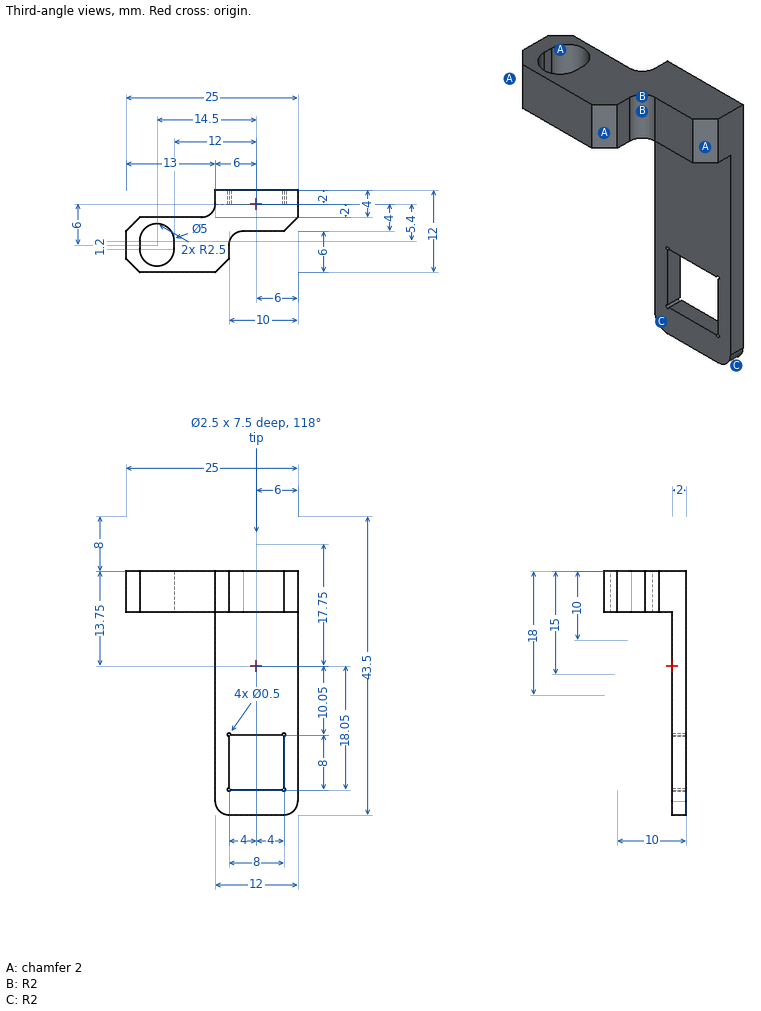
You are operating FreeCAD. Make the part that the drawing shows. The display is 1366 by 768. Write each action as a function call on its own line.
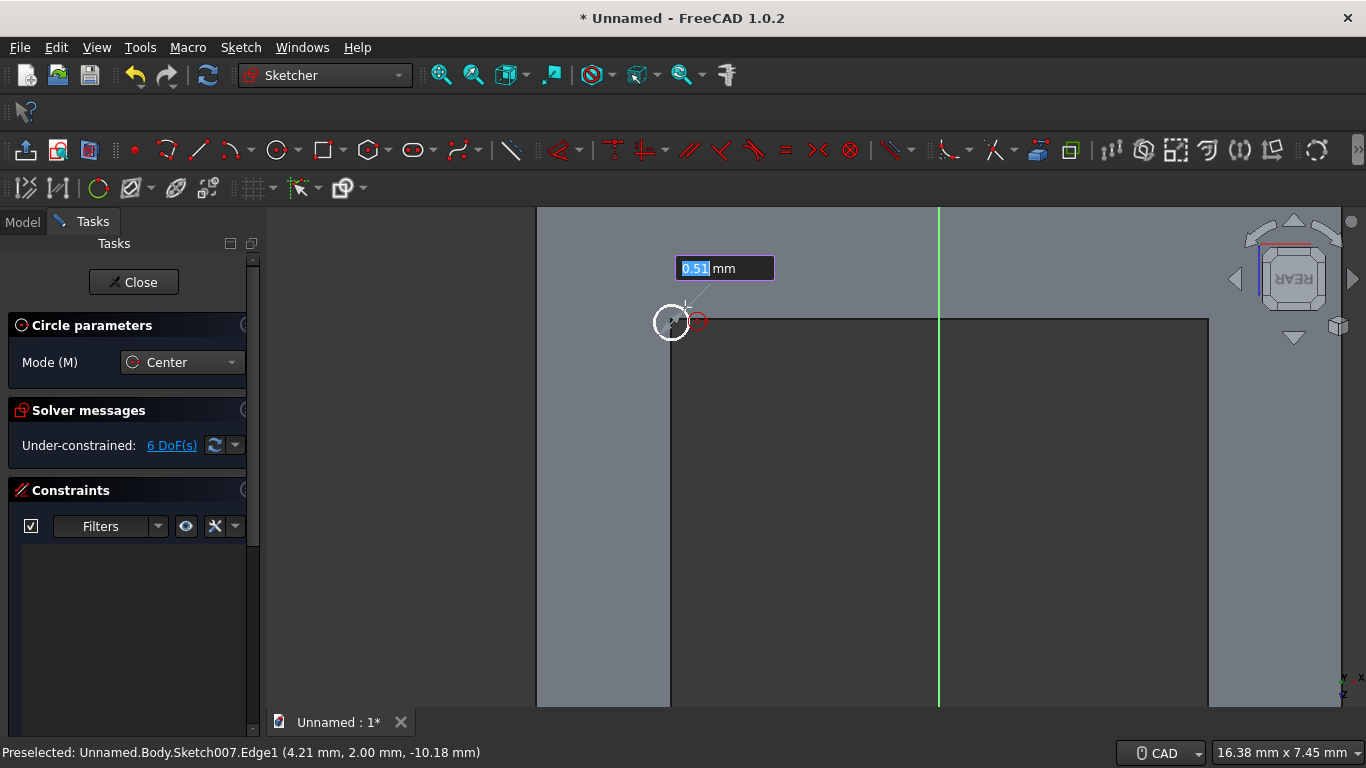
click(683, 307)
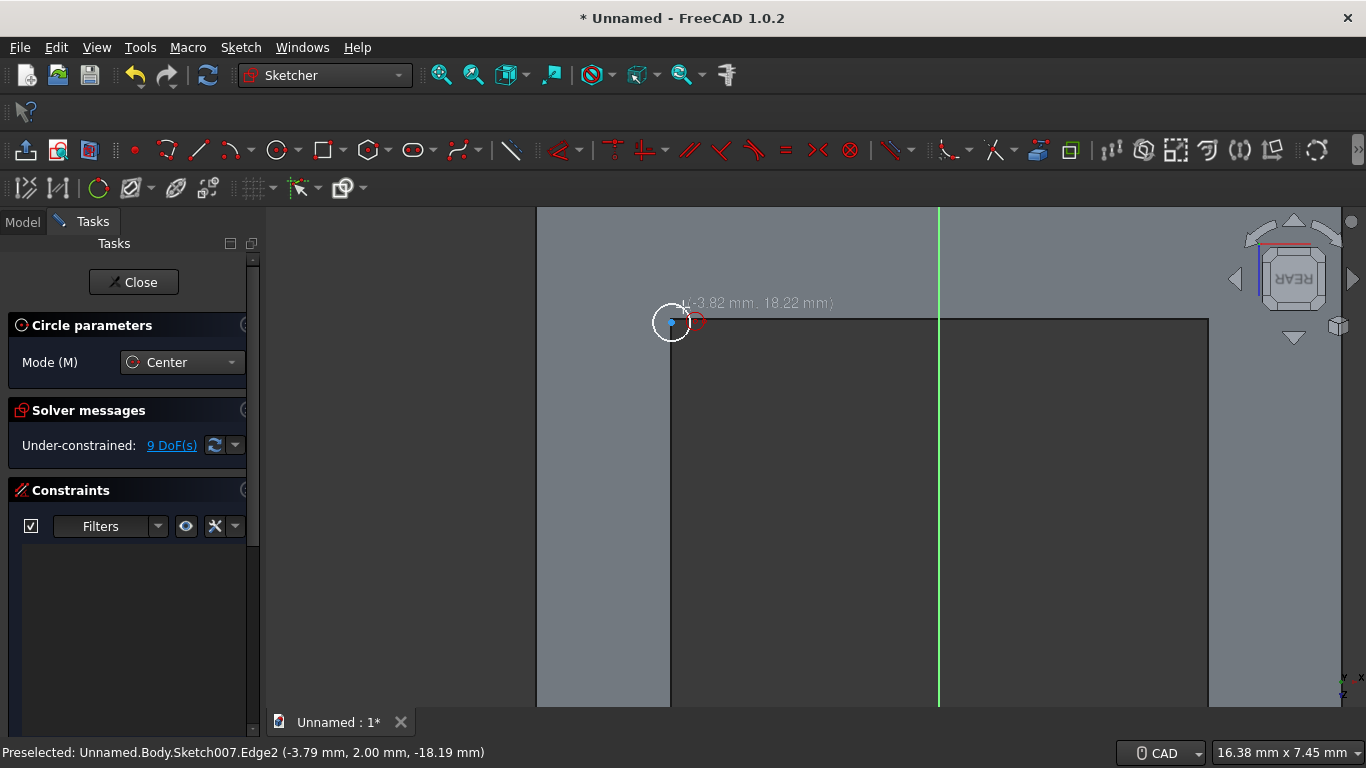
scroll(685, 306, down, 7)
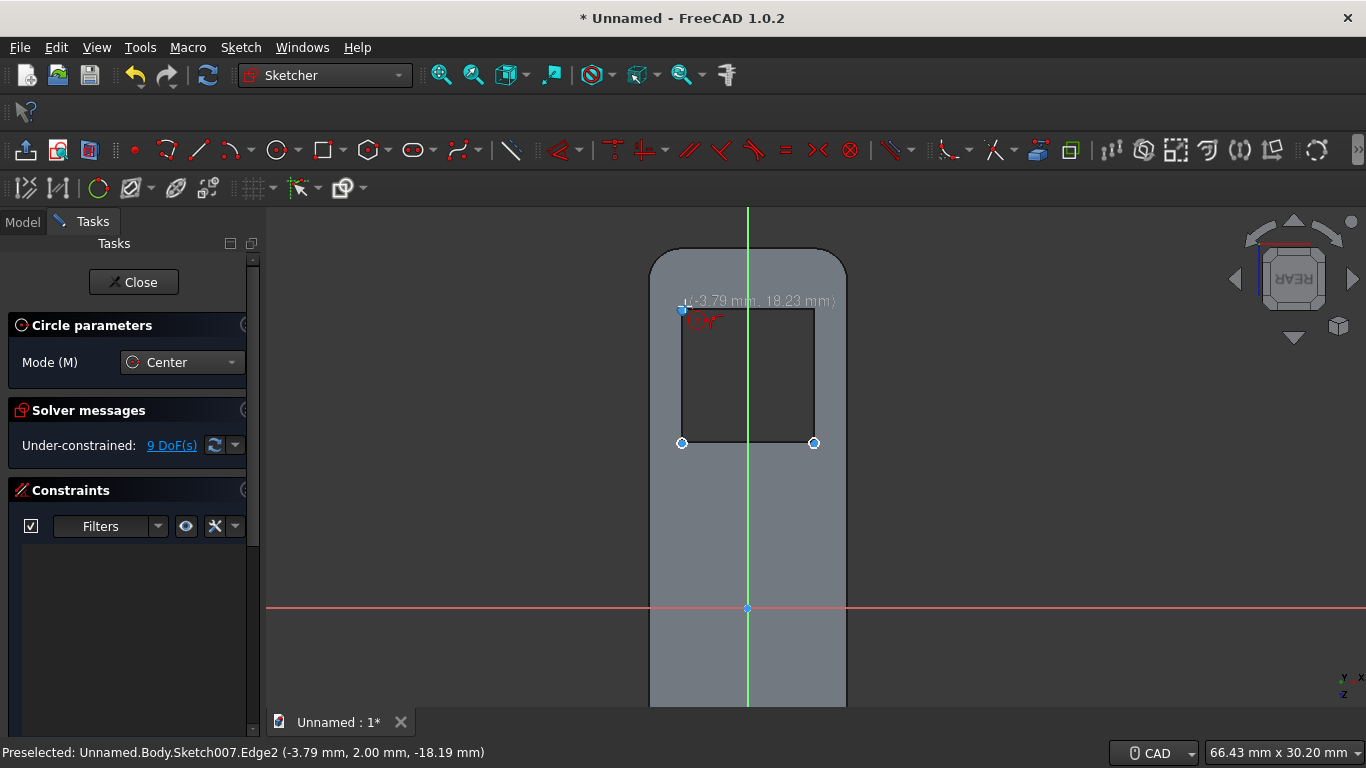
scroll(814, 309, up, 9)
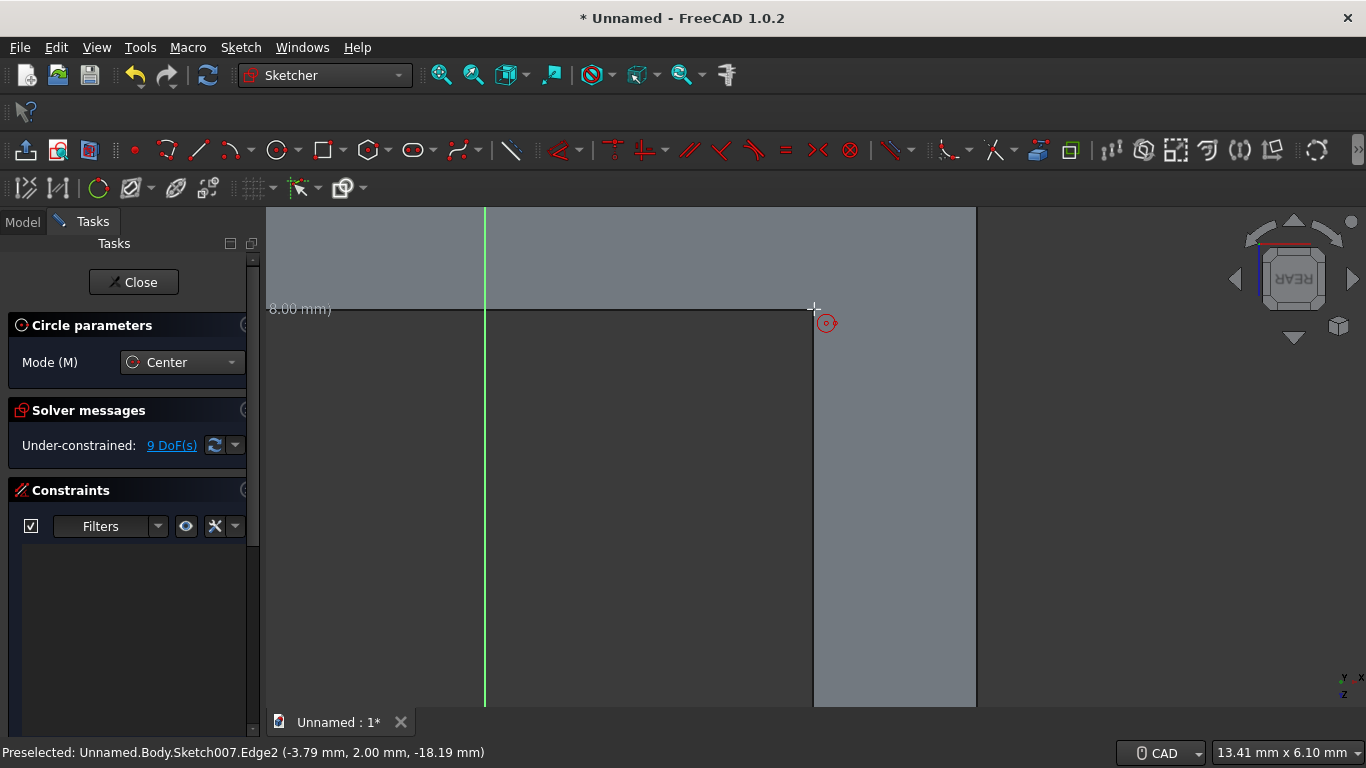
scroll(814, 309, down, 9)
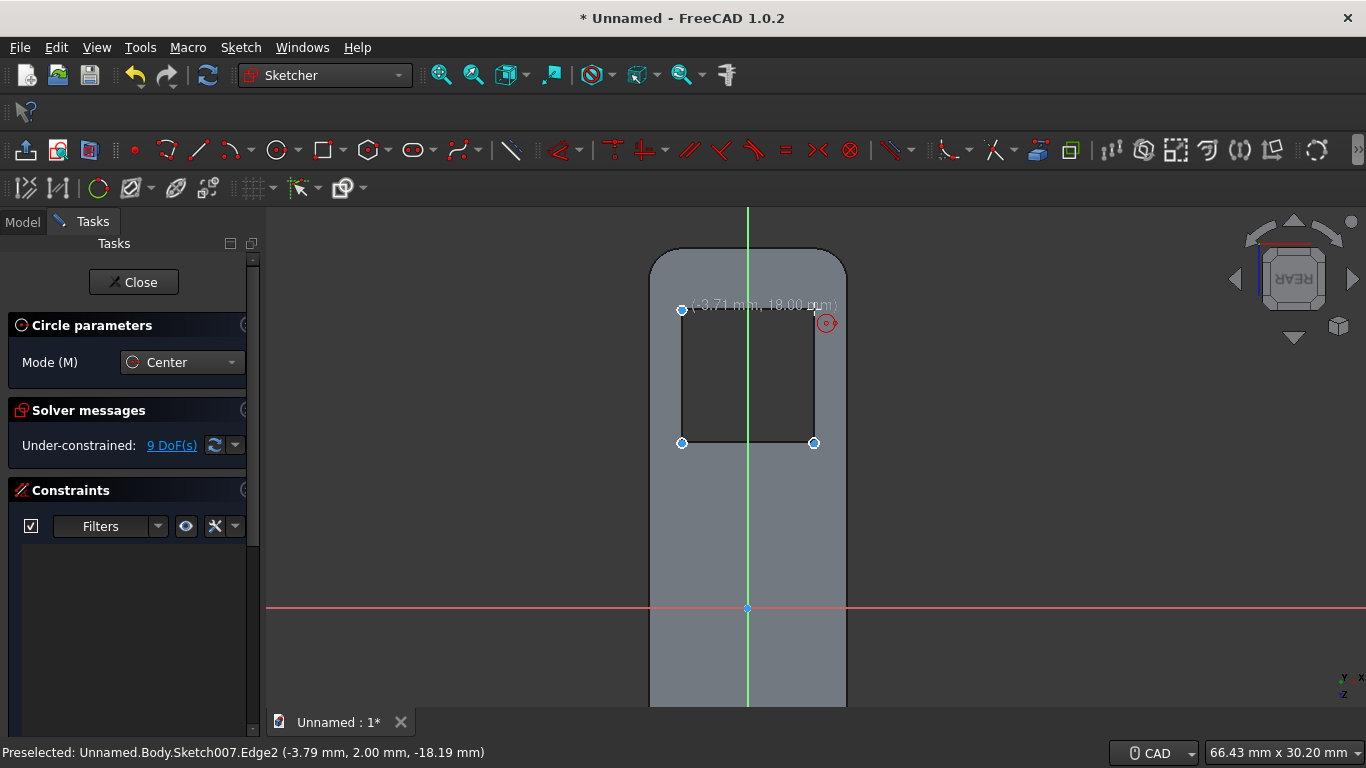
click(814, 309)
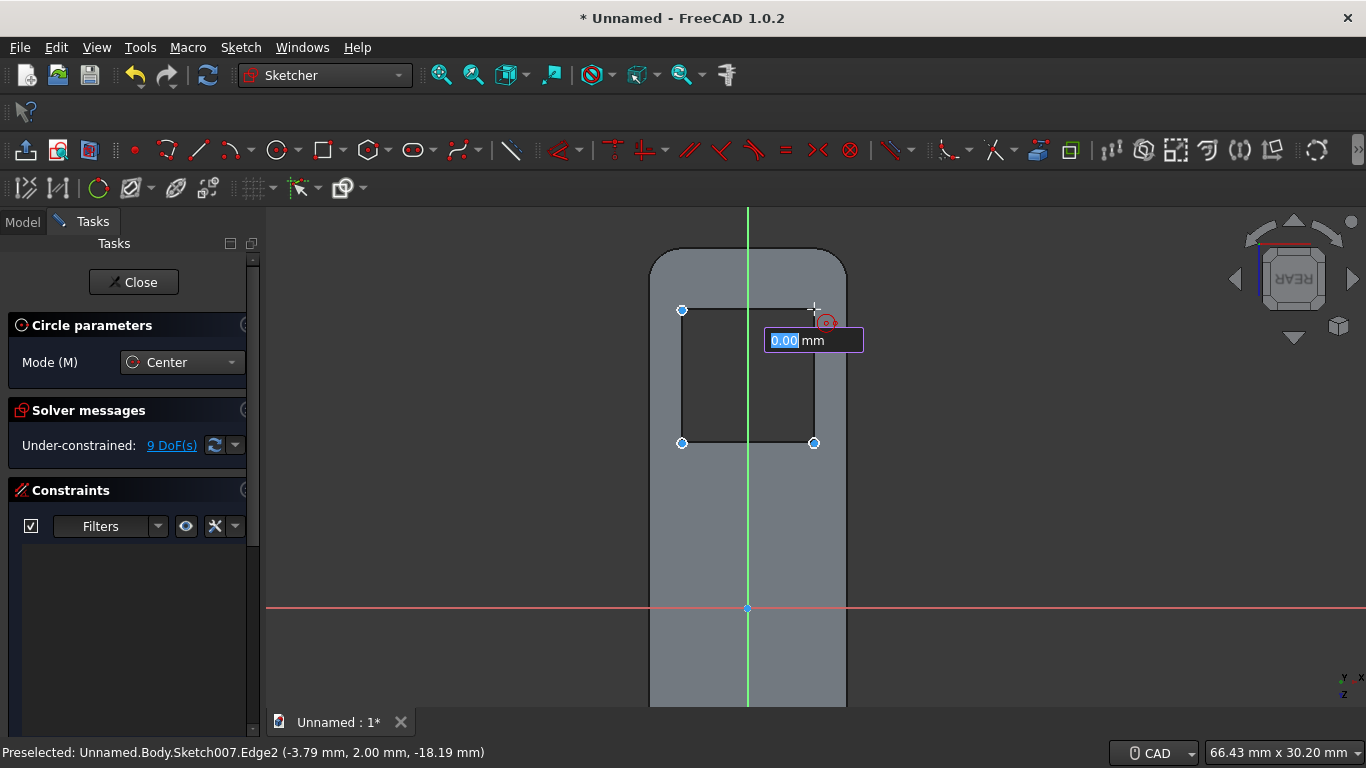
scroll(817, 307, up, 7)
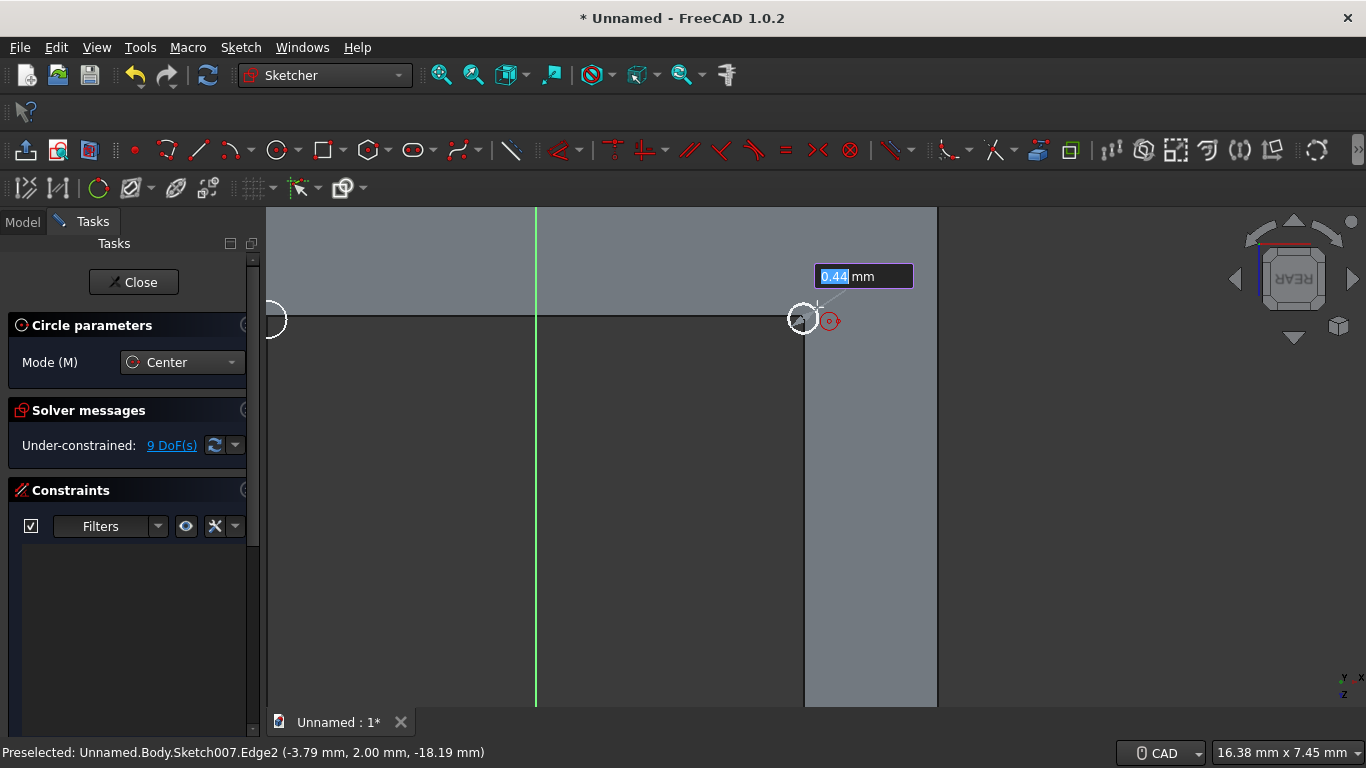
click(816, 304)
key(Escape)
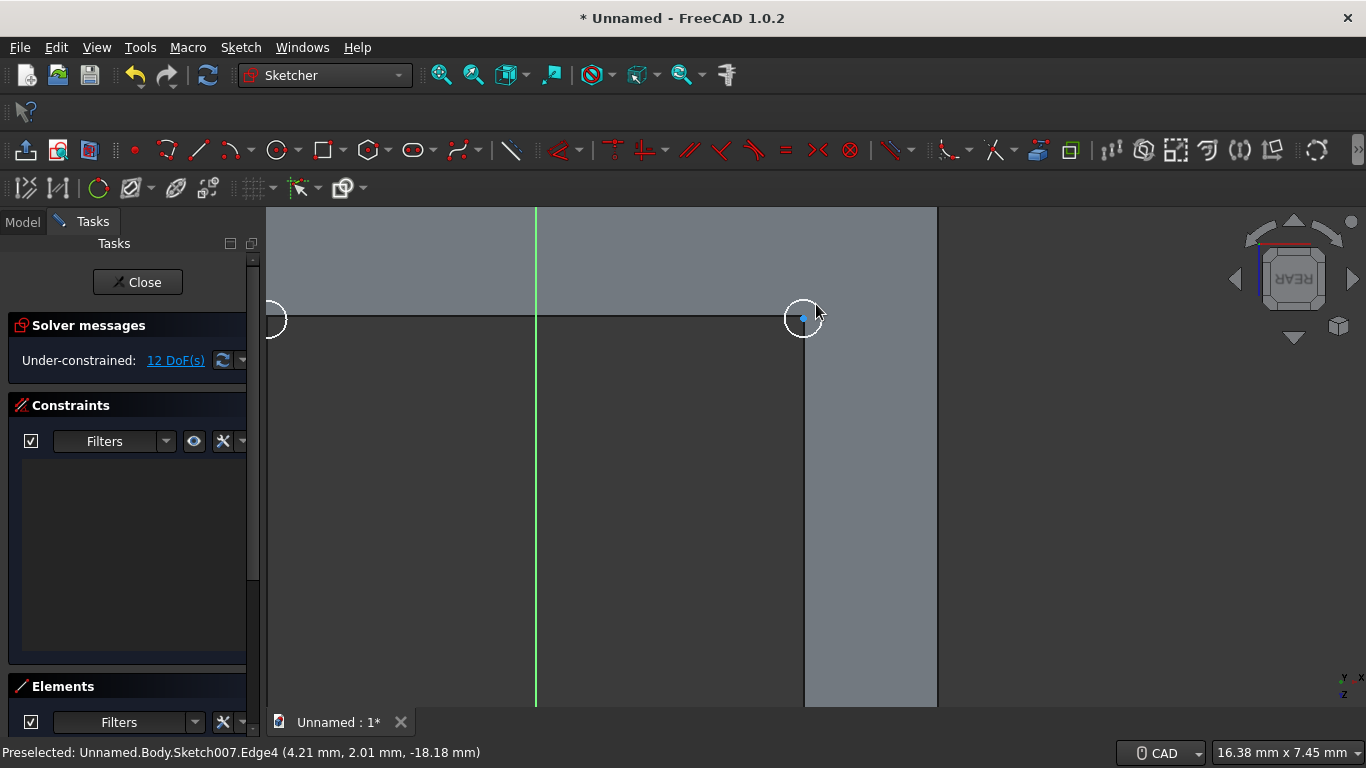
scroll(817, 307, down, 7)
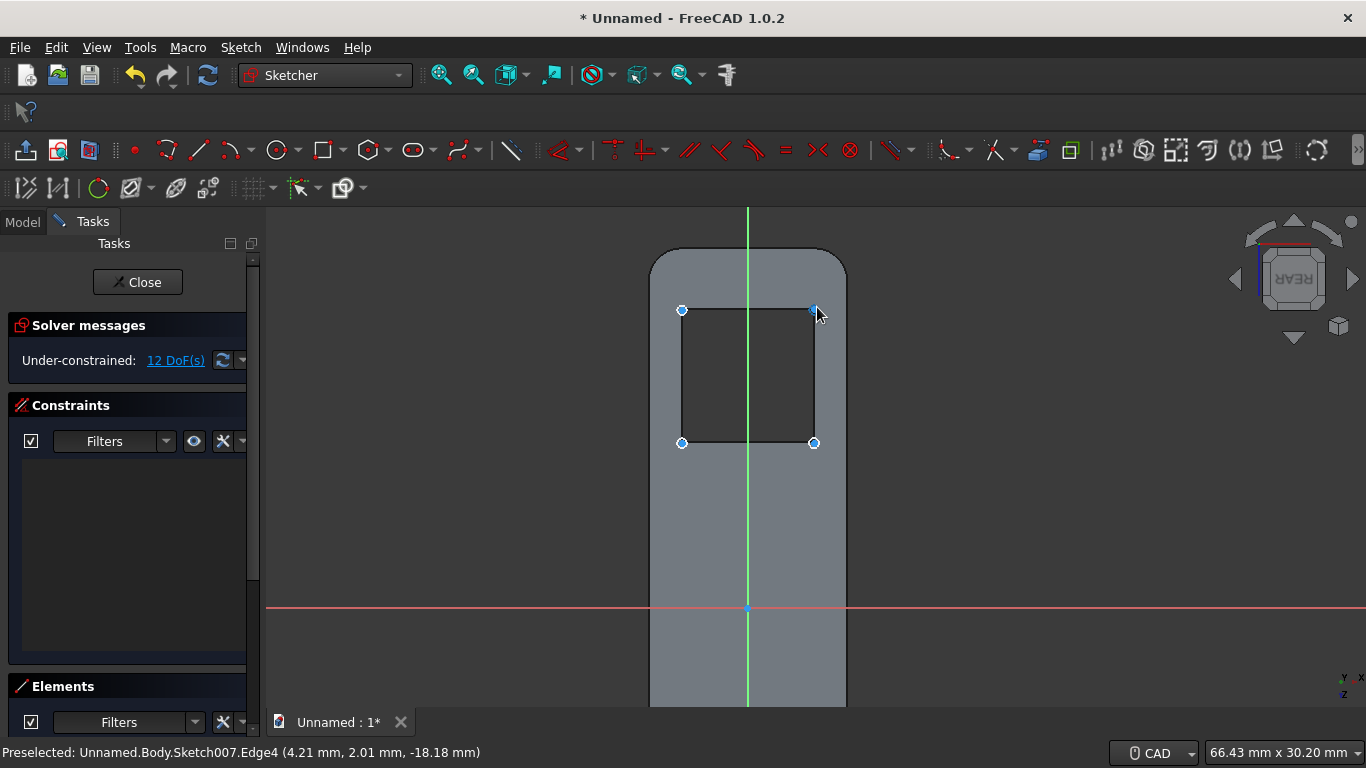
scroll(685, 440, up, 6)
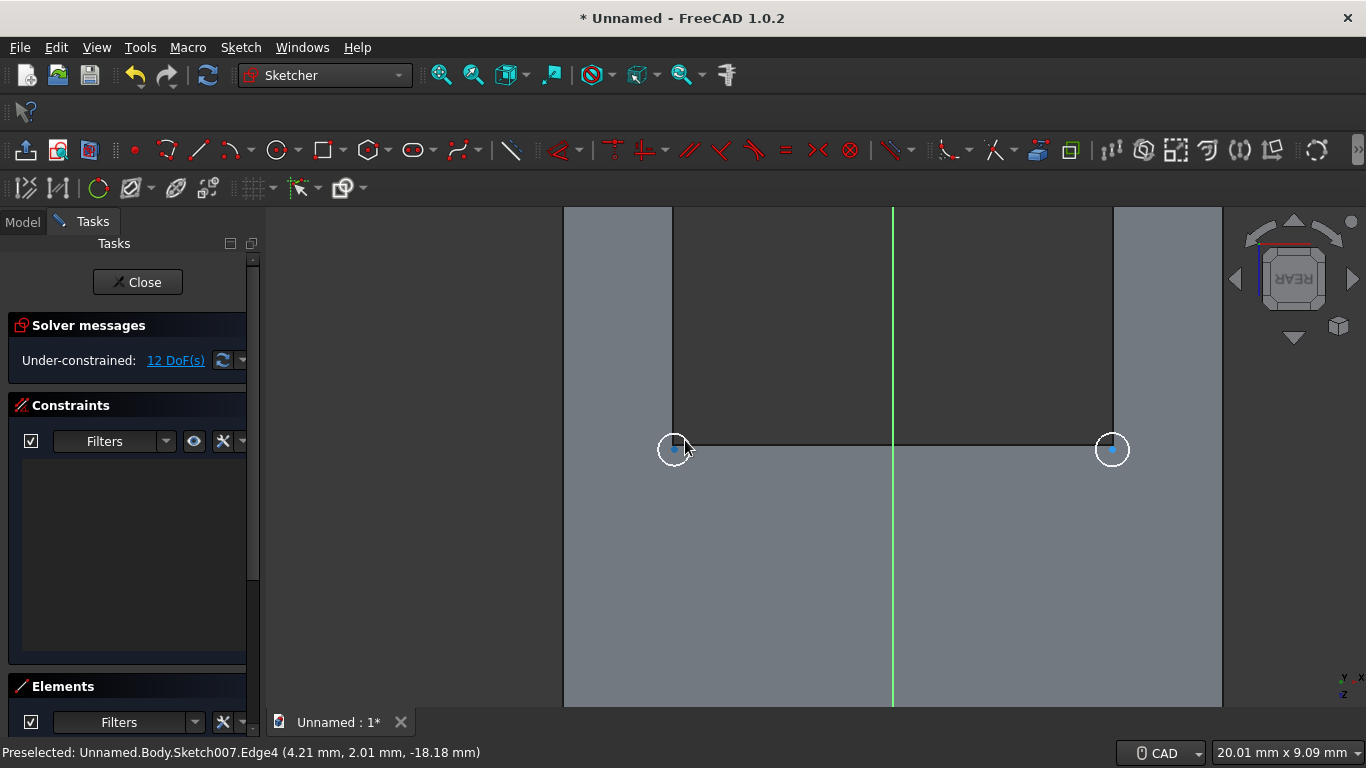
click(685, 438)